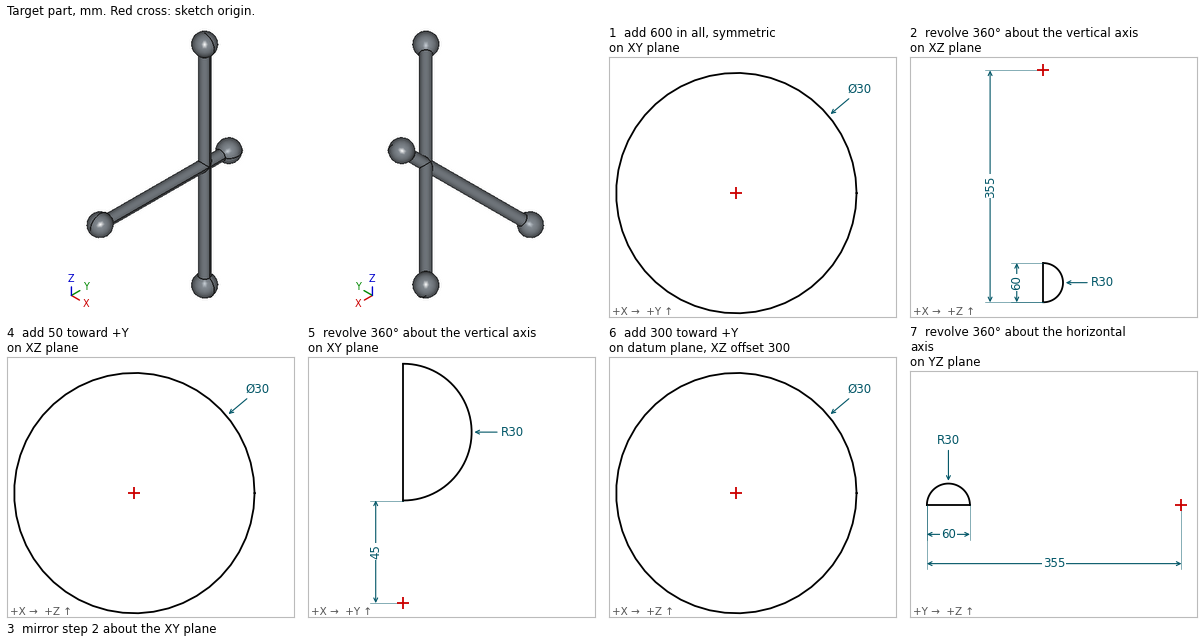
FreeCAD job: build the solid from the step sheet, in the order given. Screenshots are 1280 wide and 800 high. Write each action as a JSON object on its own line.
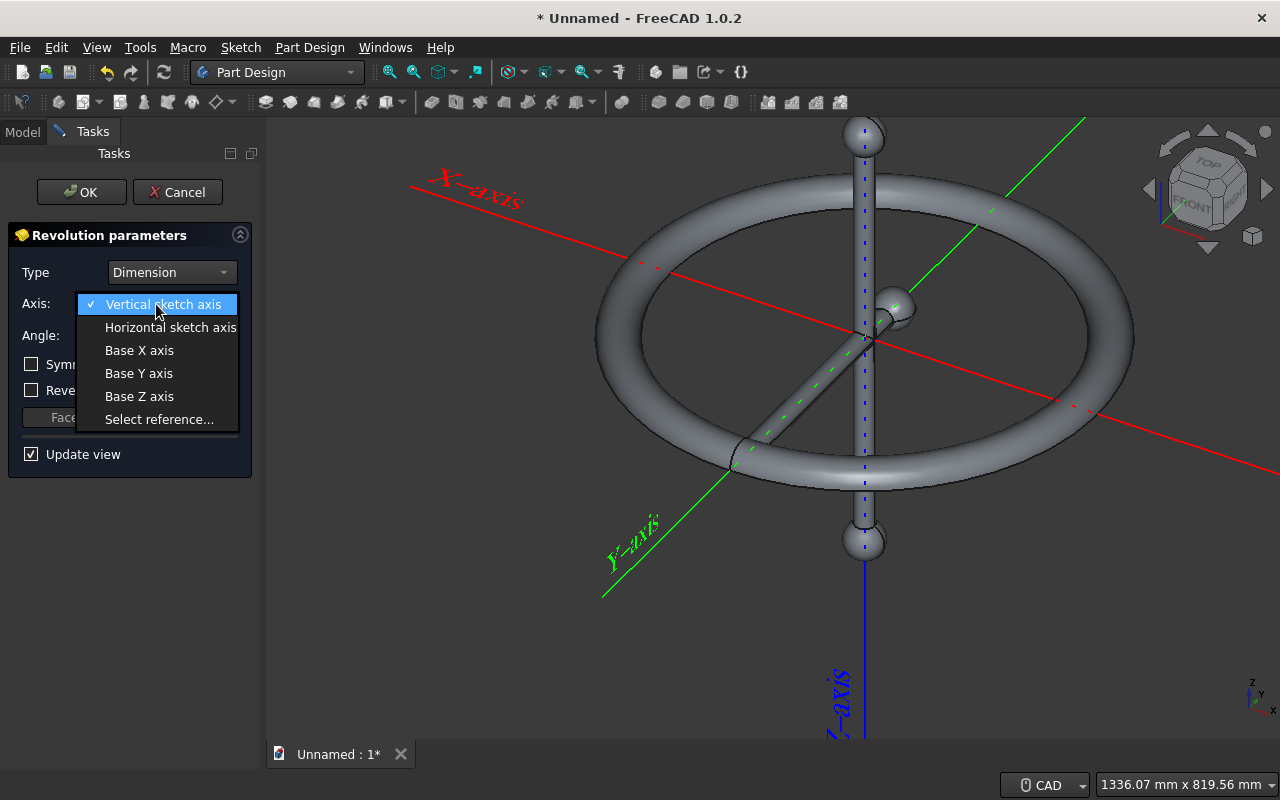
{"action": "left_click", "coordinate": [156, 328]}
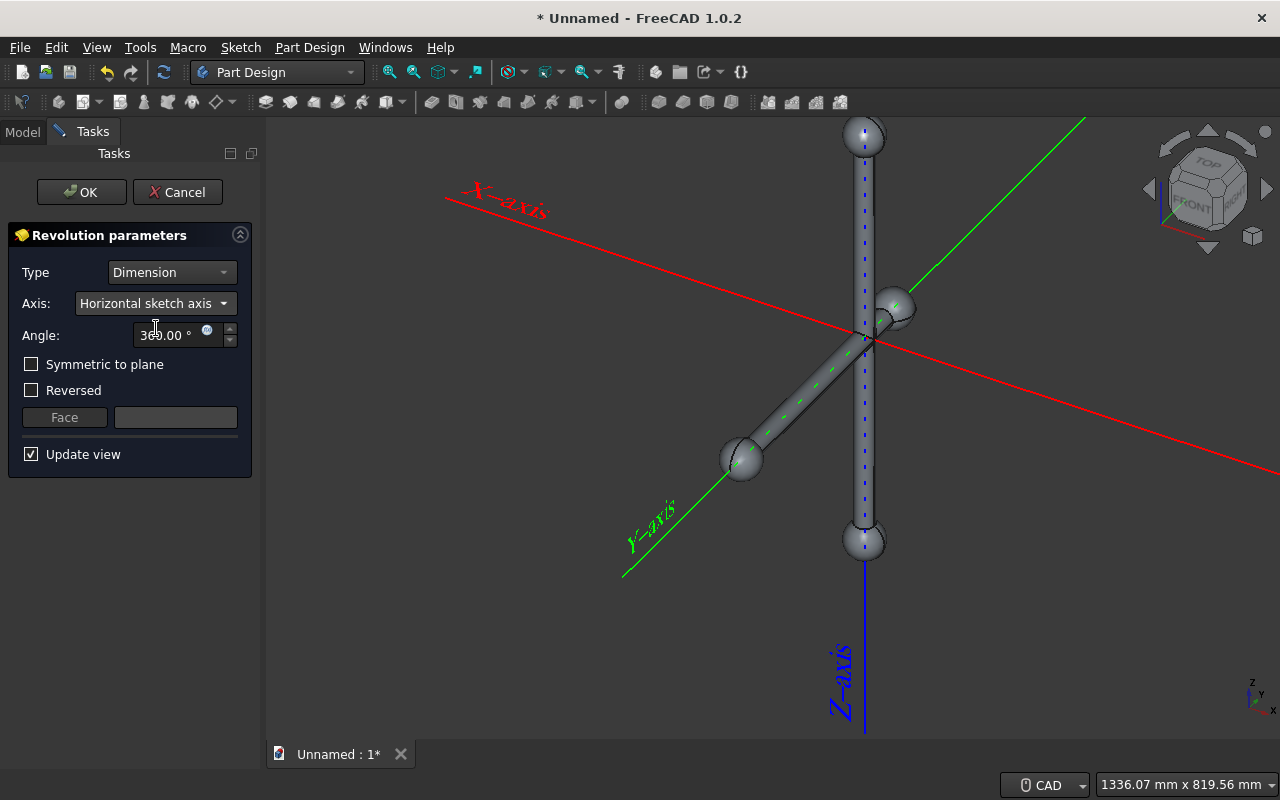
{"action": "left_click", "coordinate": [82, 192]}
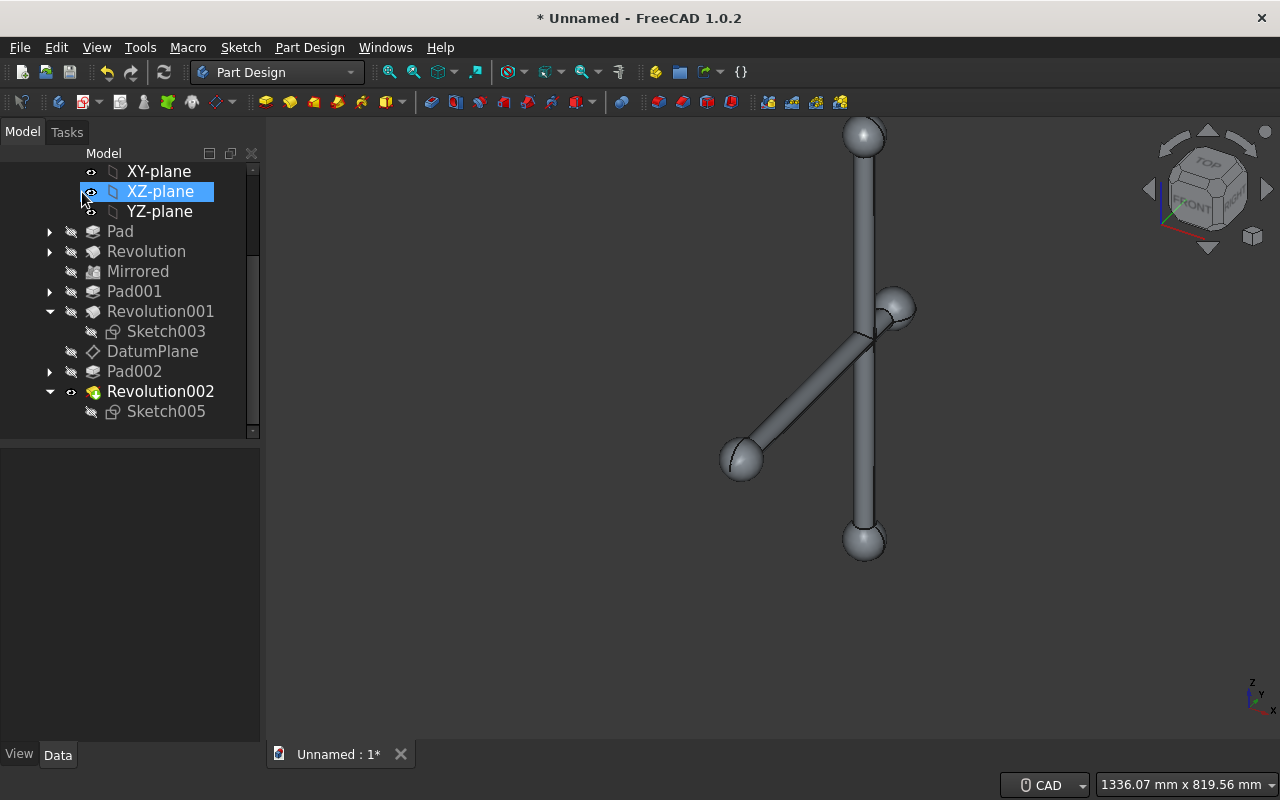
{"action": "key", "text": "0"}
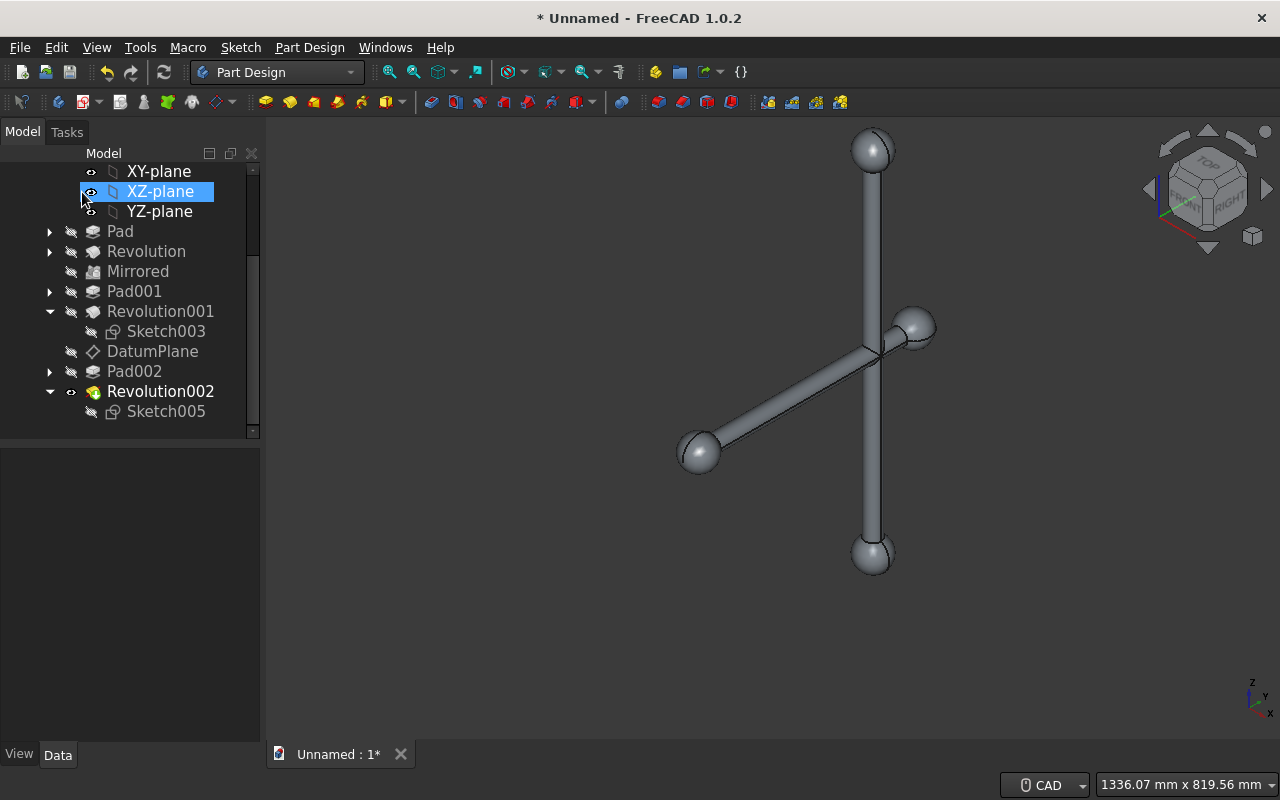
{"action": "left_click", "coordinate": [390, 72]}